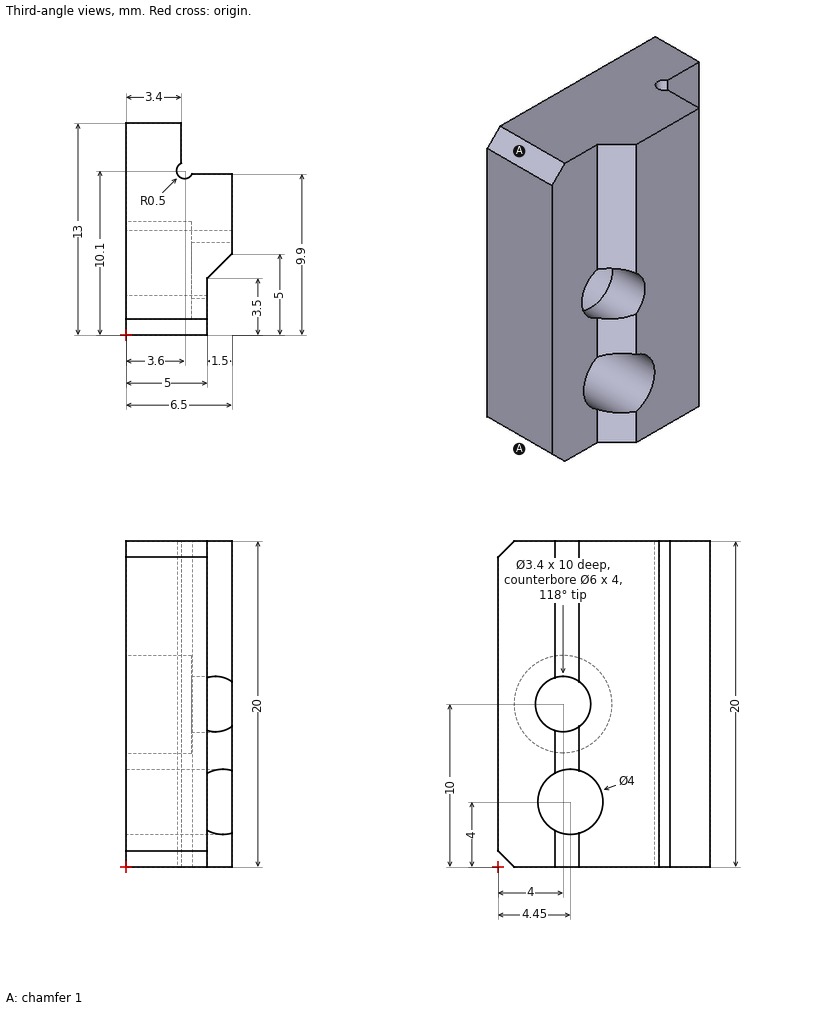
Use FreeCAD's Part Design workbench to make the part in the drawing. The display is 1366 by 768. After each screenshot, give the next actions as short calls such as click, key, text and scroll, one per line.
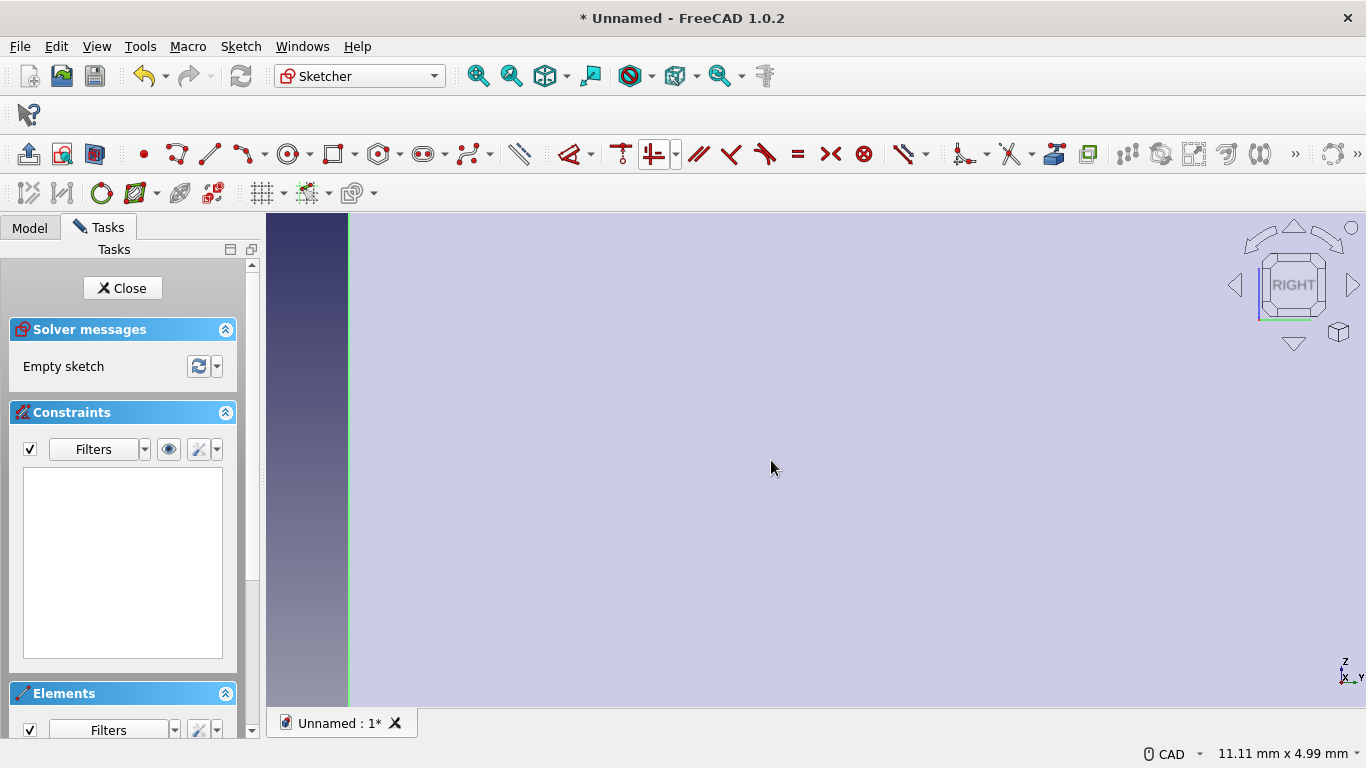
click(288, 154)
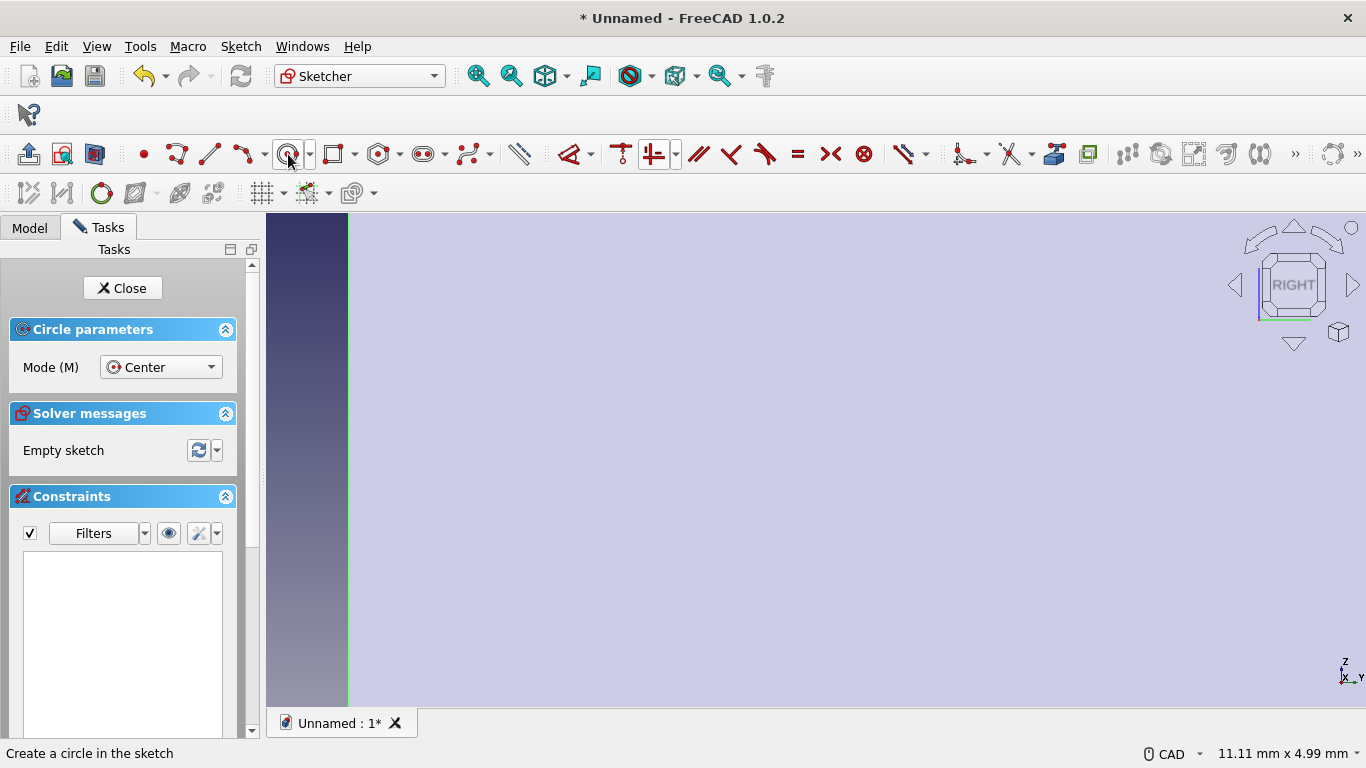
click(745, 458)
click(864, 339)
key(Escape)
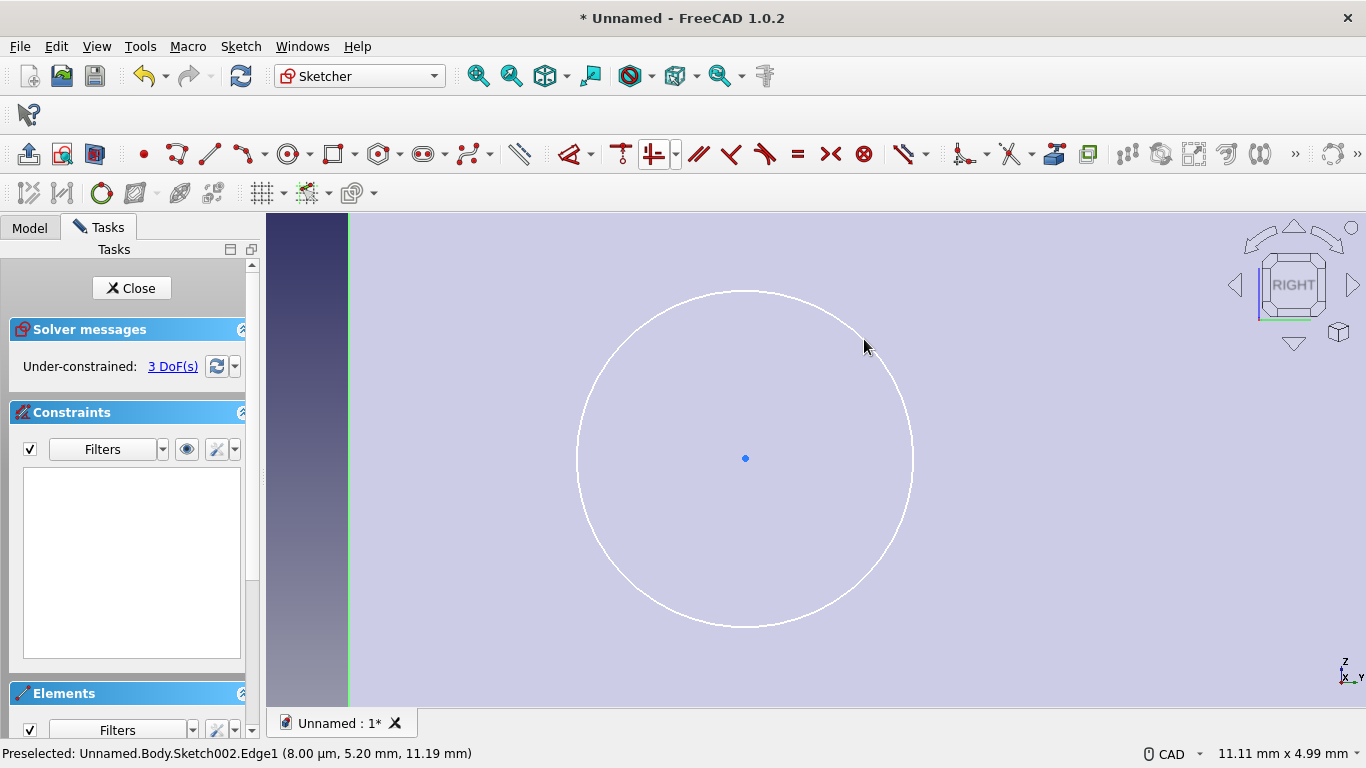
click(568, 154)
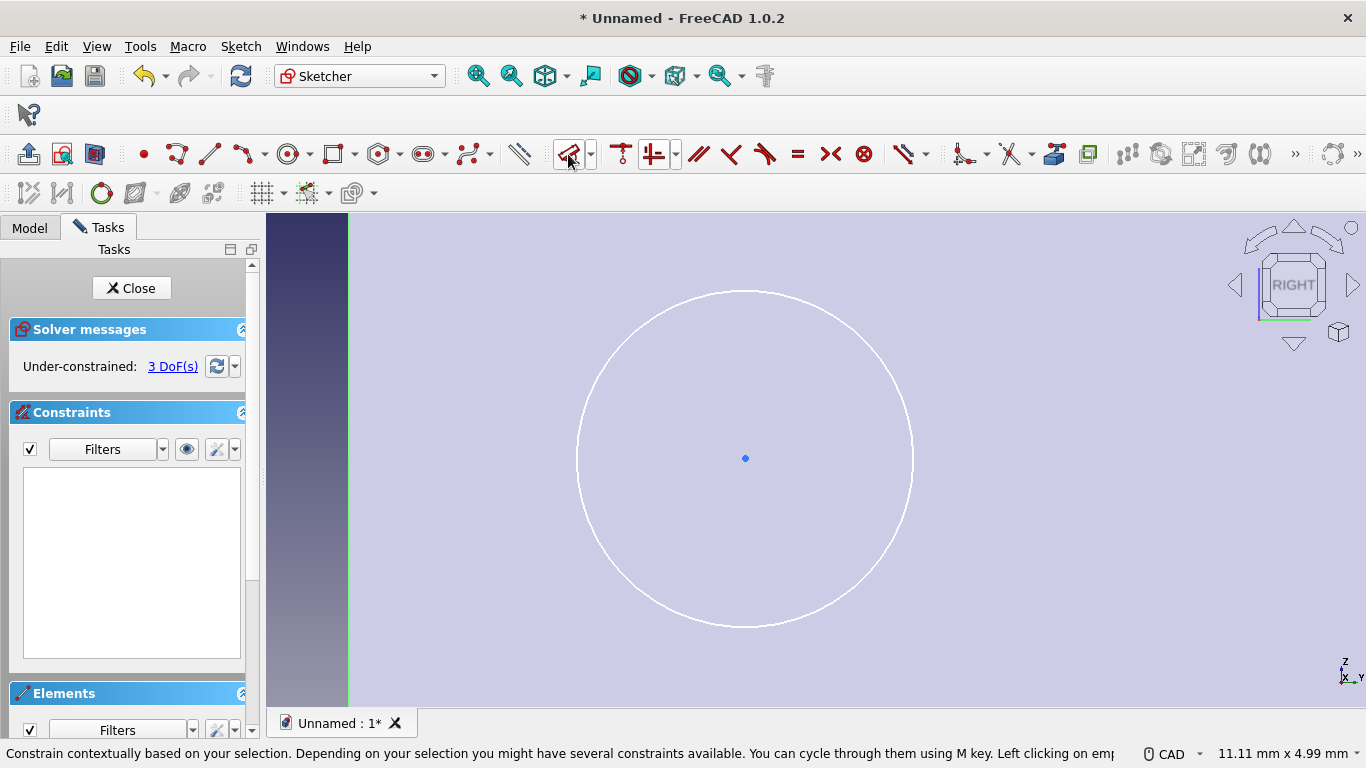
click(864, 340)
click(887, 317)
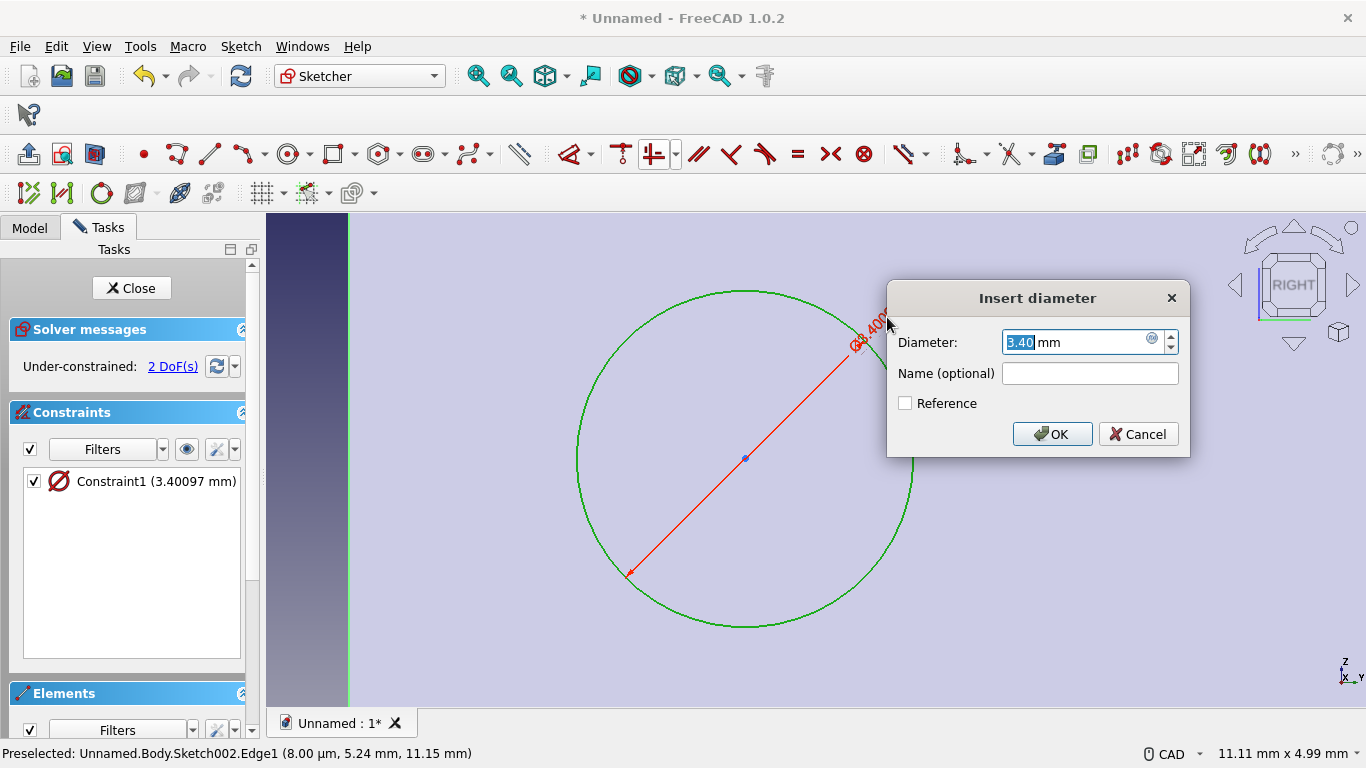
text(3.4)
key(Return)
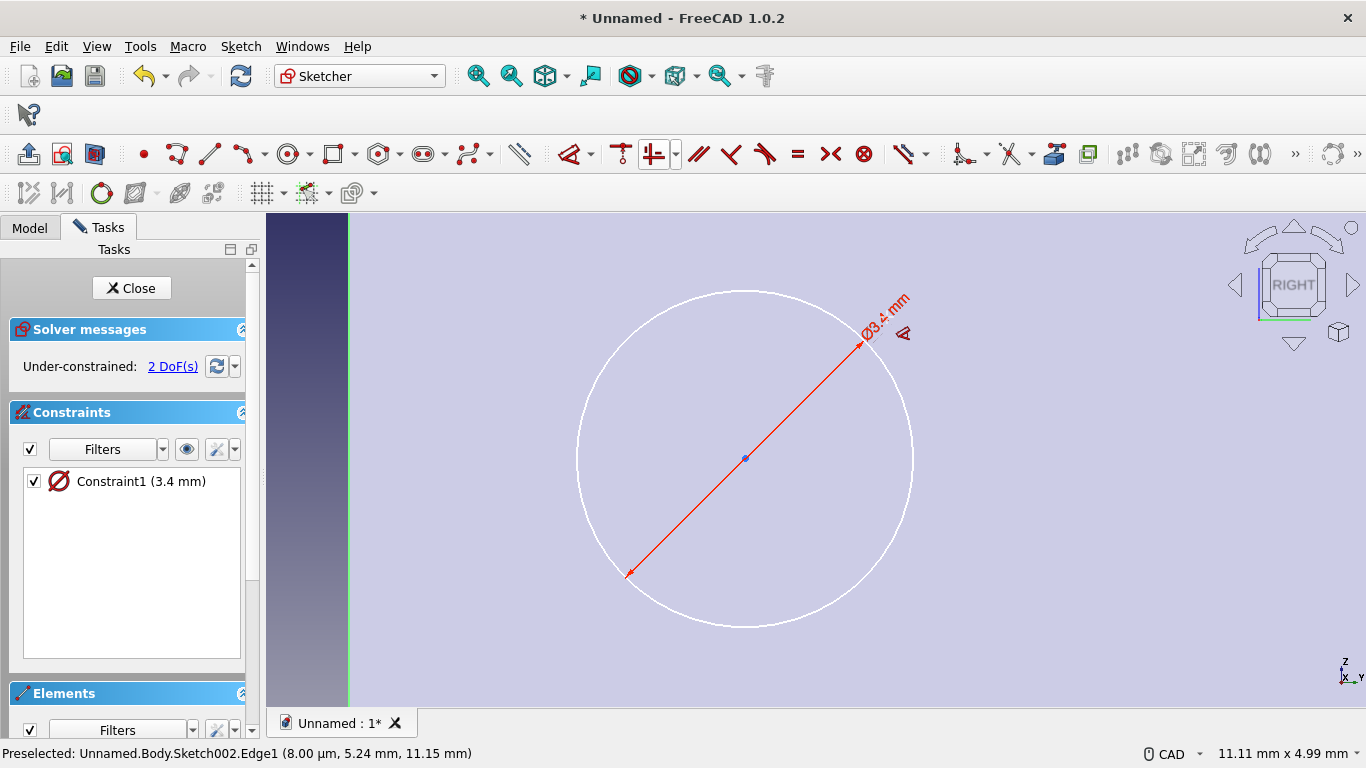
click(745, 459)
click(547, 425)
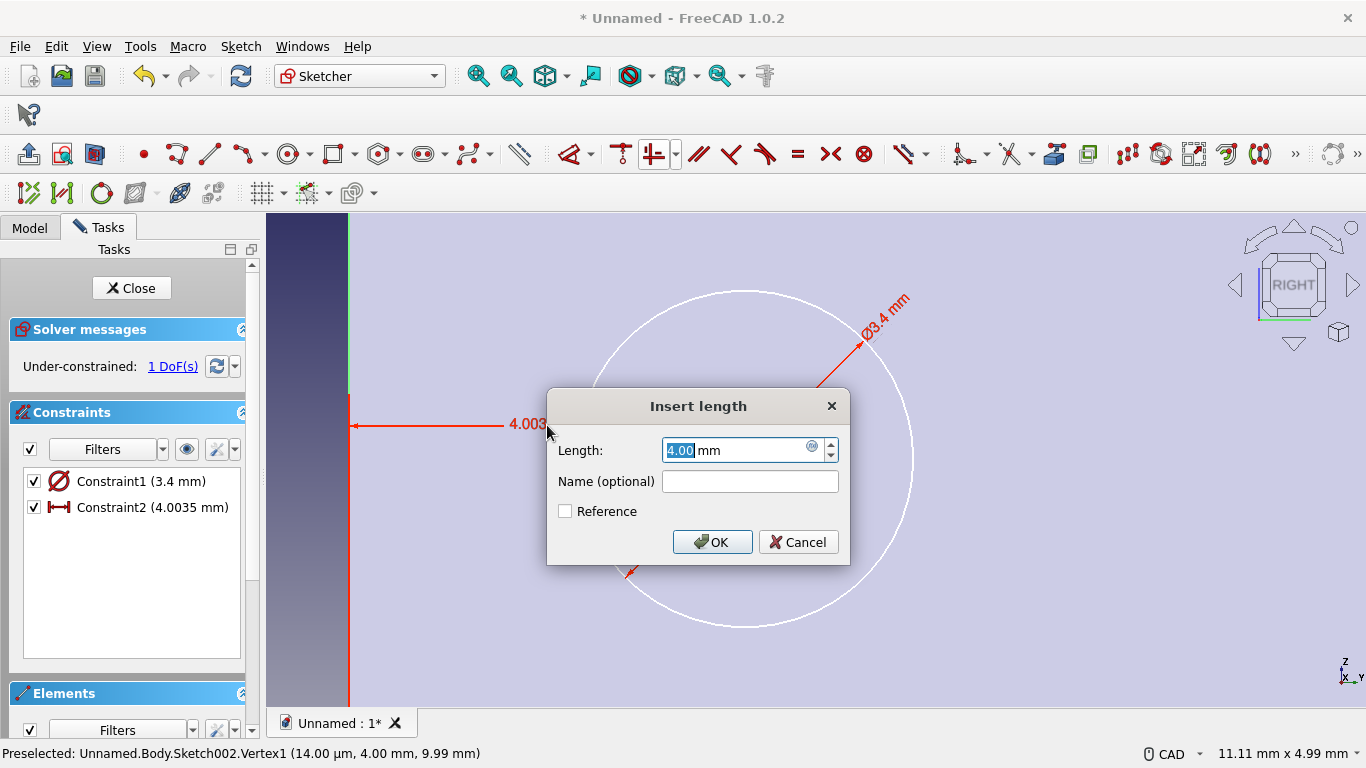
text(4)
key(Return)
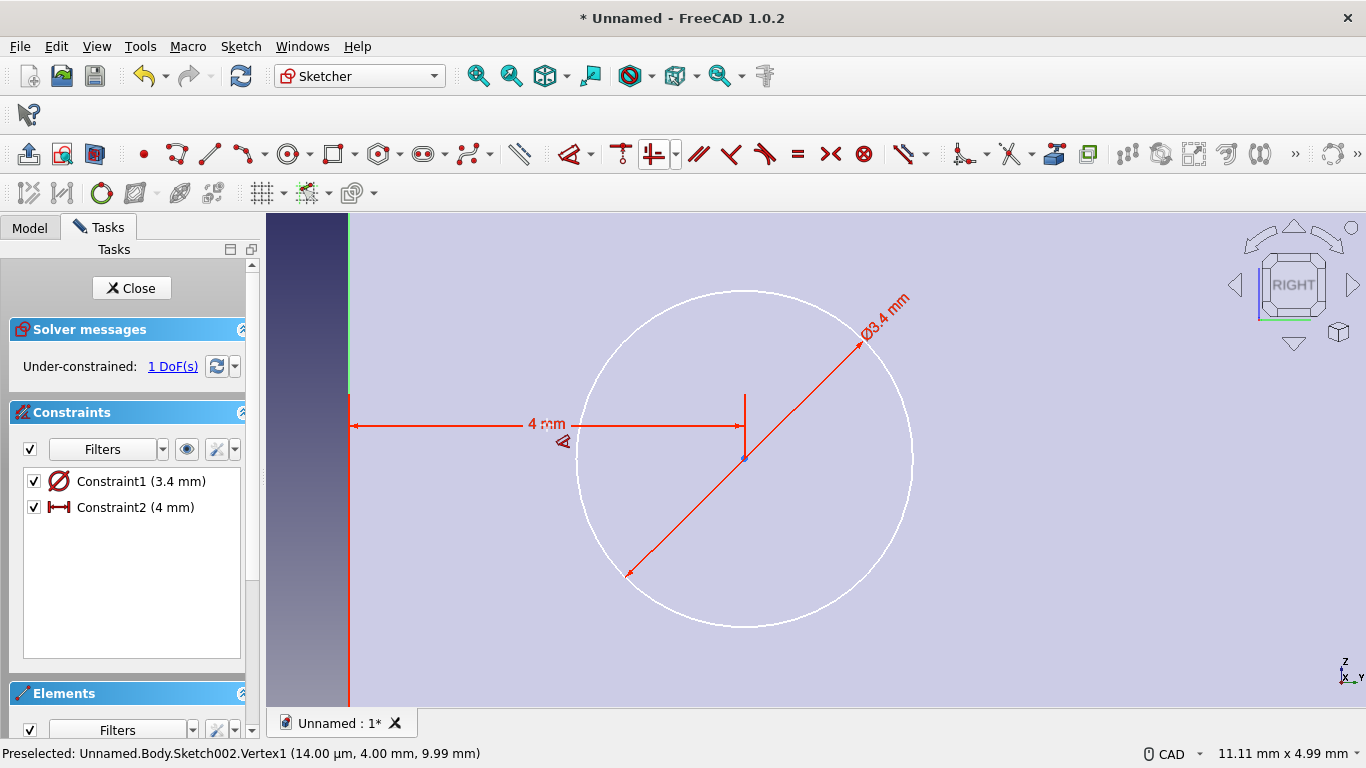
click(745, 459)
click(315, 569)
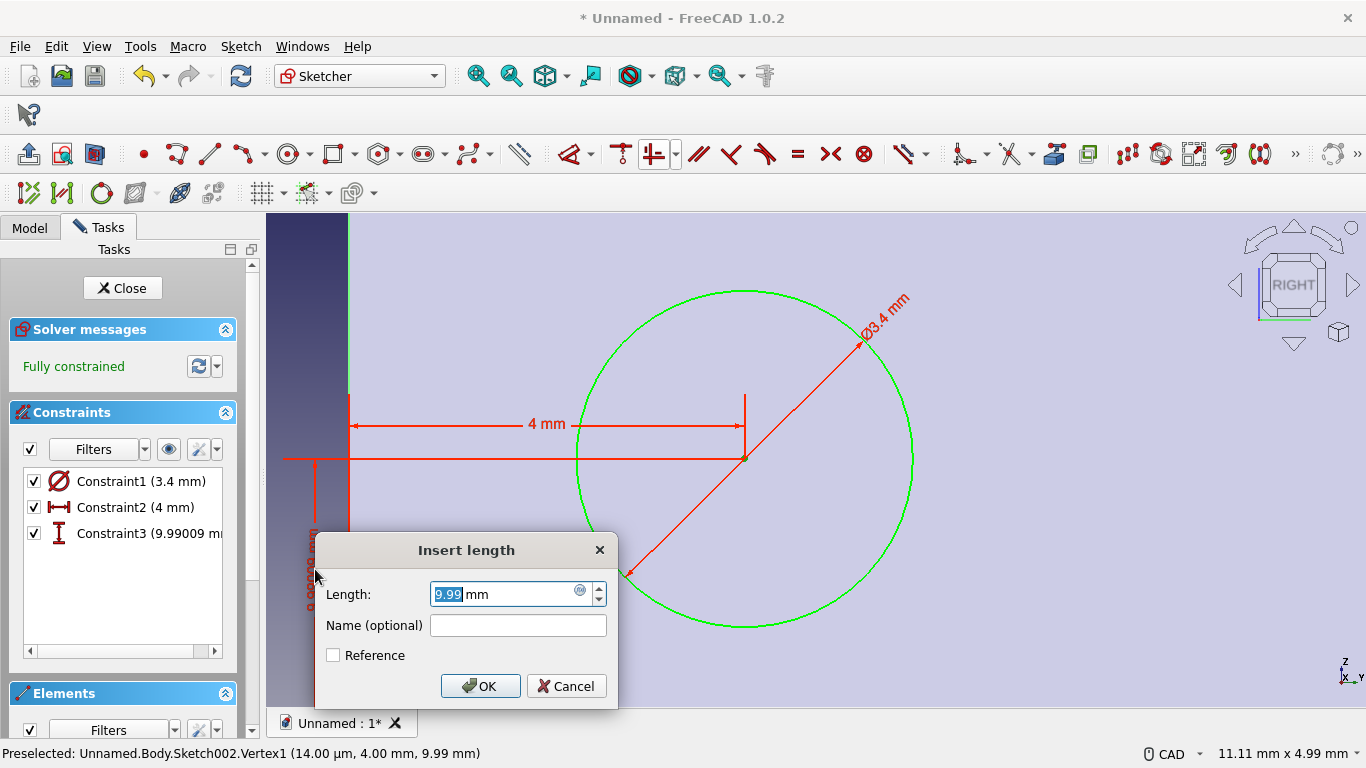
text(10)
key(Return)
key(Escape)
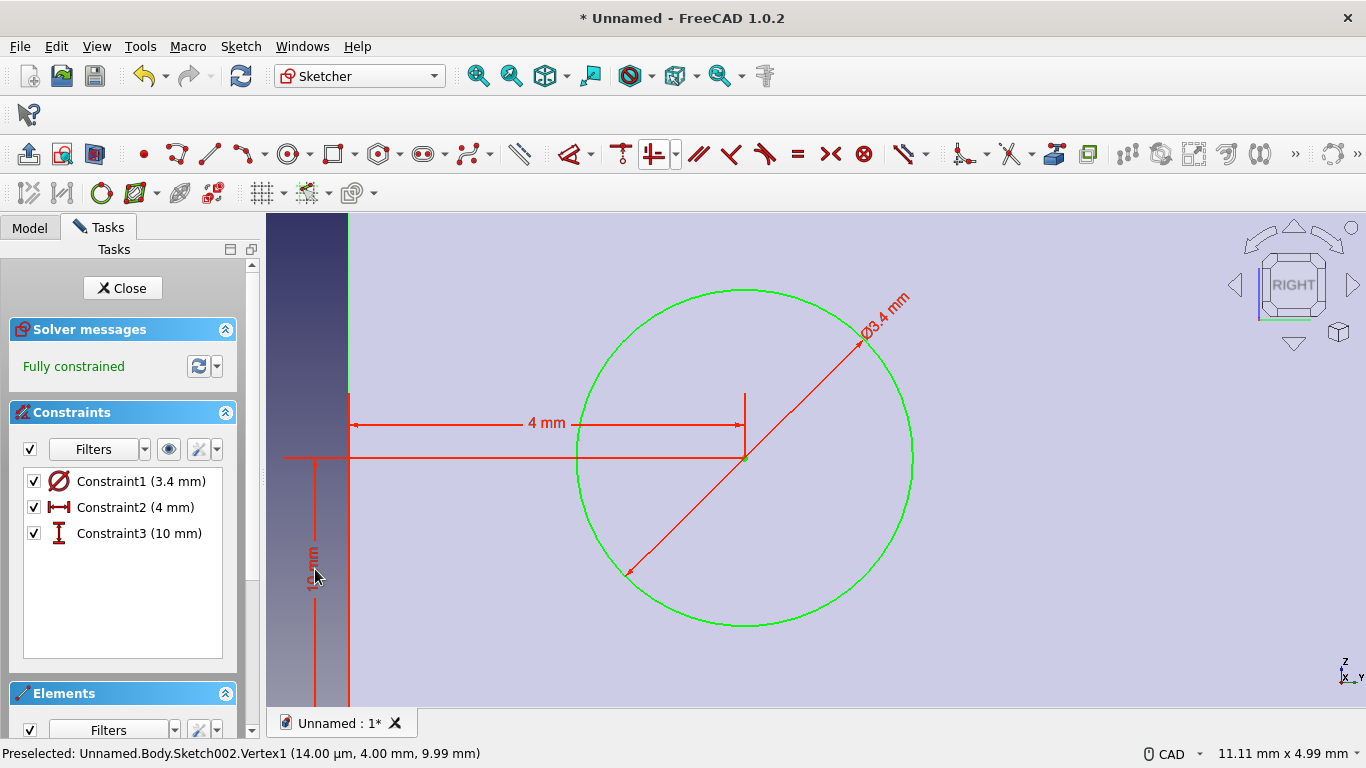
click(123, 288)